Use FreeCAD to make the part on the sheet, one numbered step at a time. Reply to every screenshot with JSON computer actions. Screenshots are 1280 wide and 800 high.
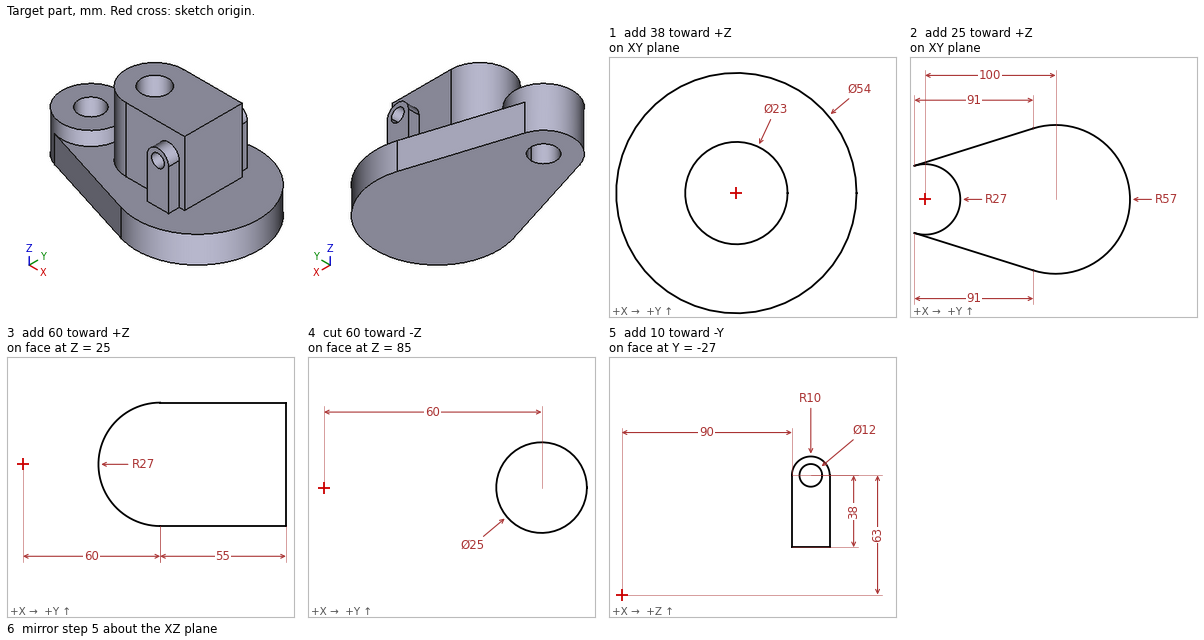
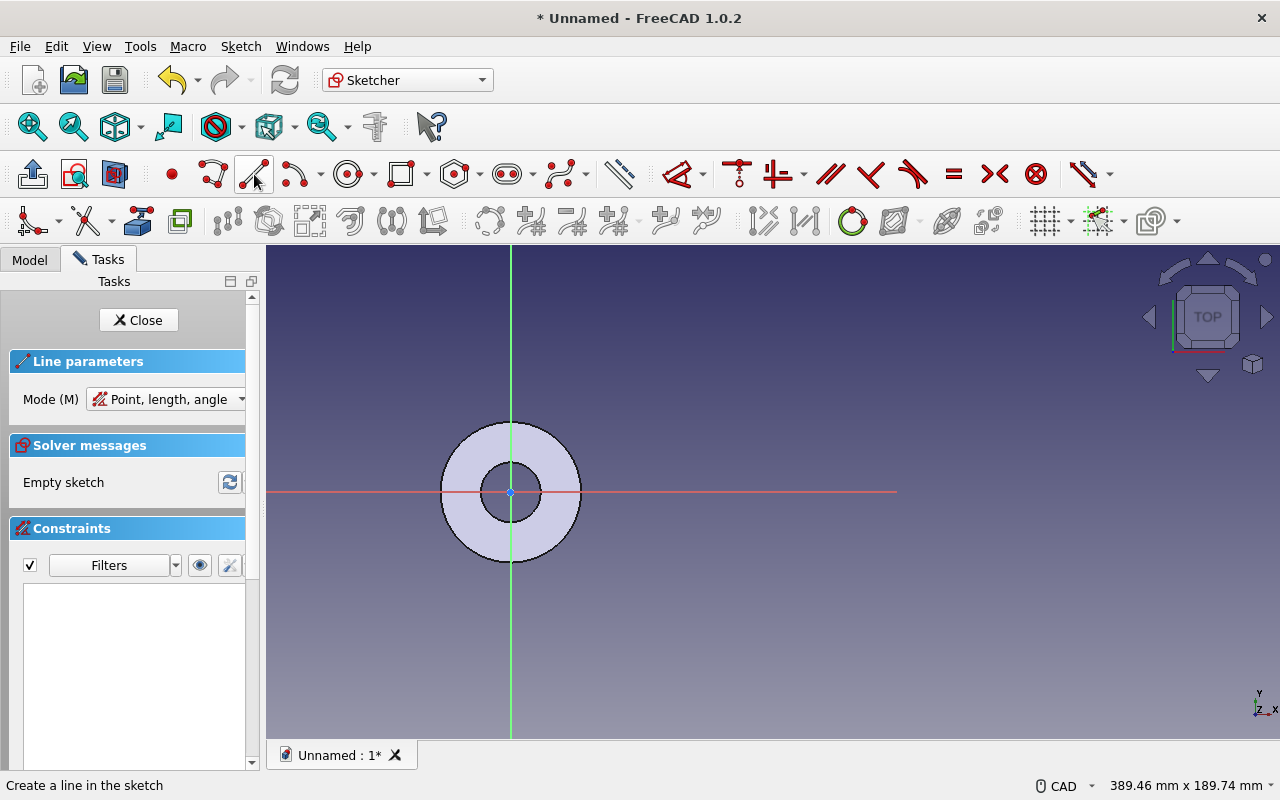
{"action": "left_click", "coordinate": [727, 351]}
{"action": "left_click", "coordinate": [490, 425]}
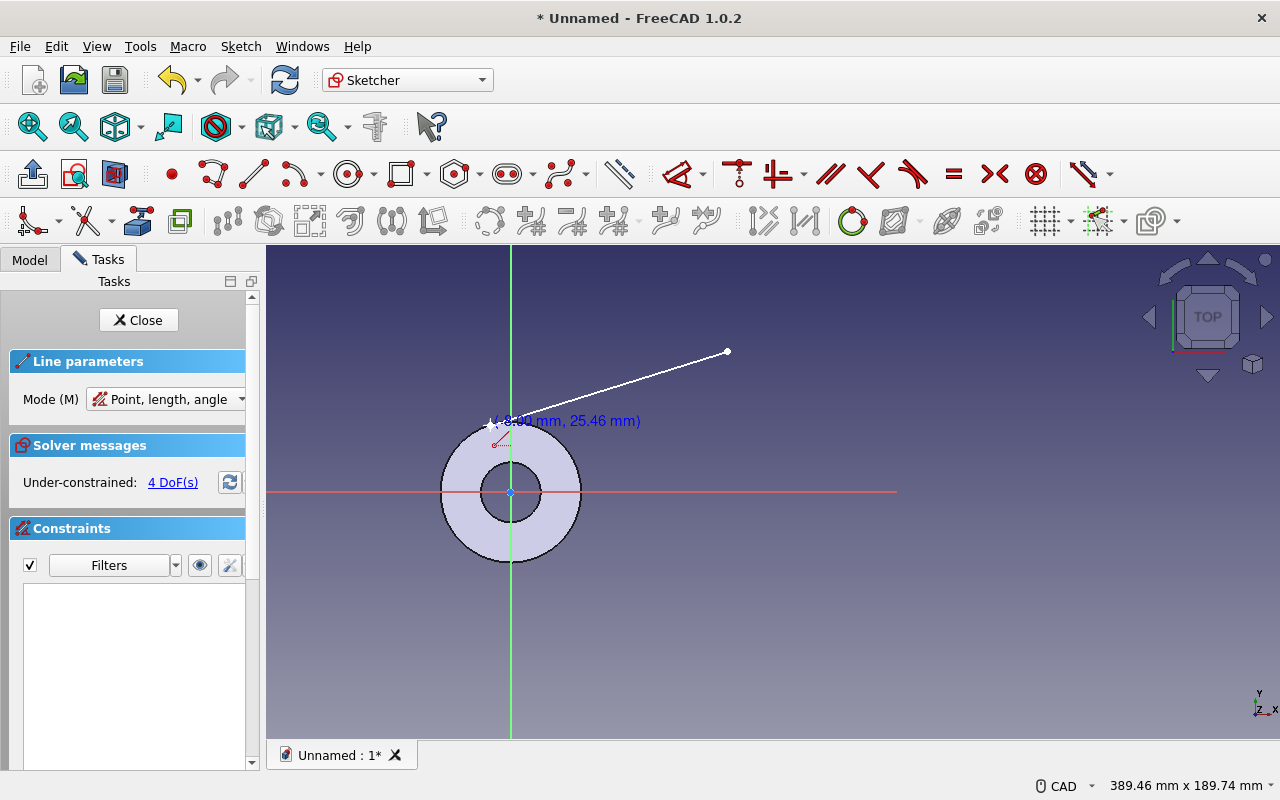
{"action": "left_click", "coordinate": [490, 559]}
{"action": "left_click", "coordinate": [727, 634]}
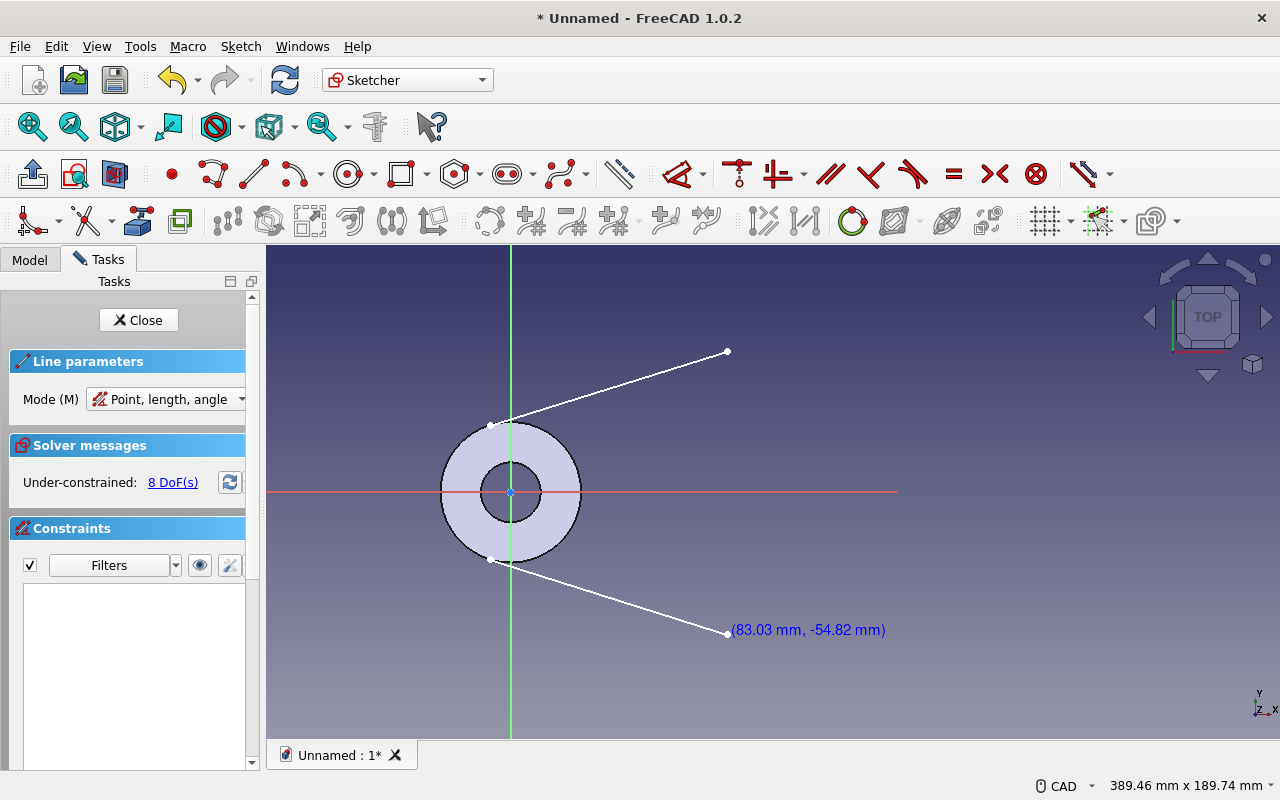
{"action": "left_click", "coordinate": [320, 174]}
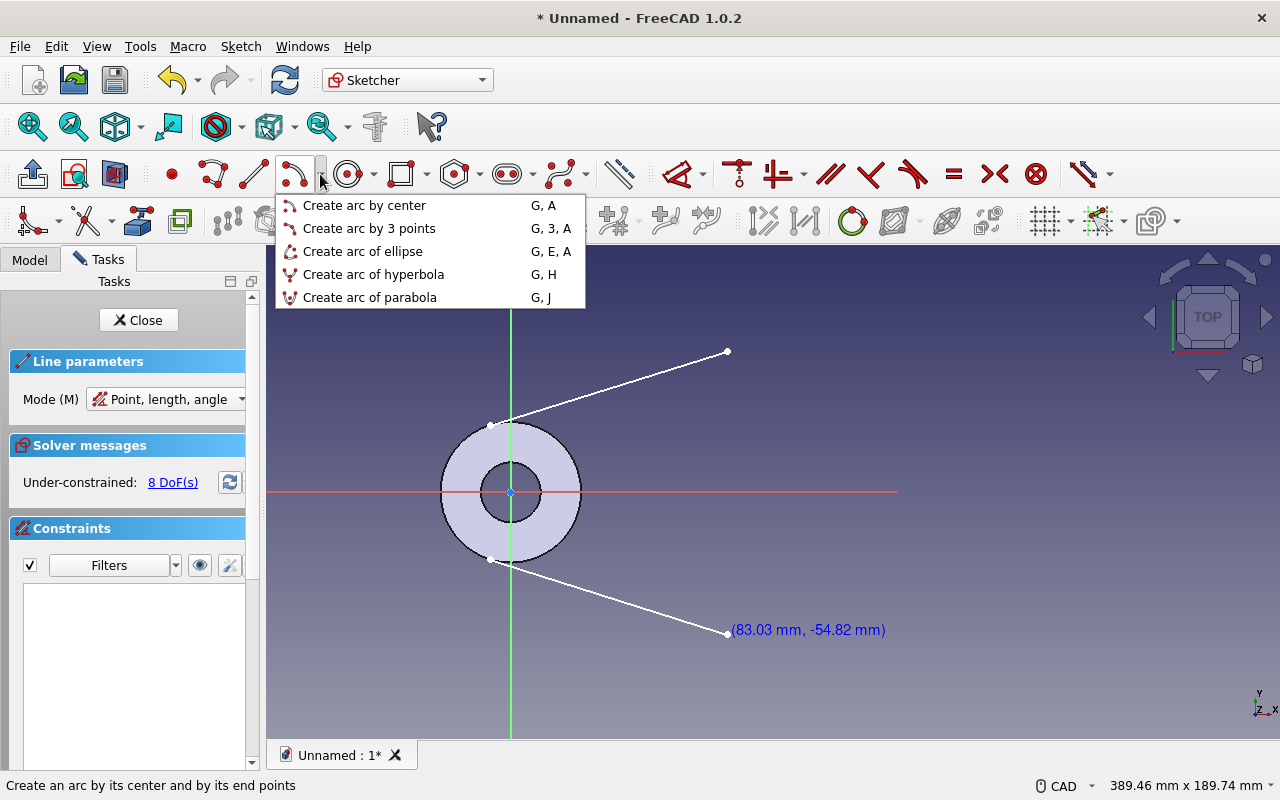
{"action": "left_click", "coordinate": [430, 228]}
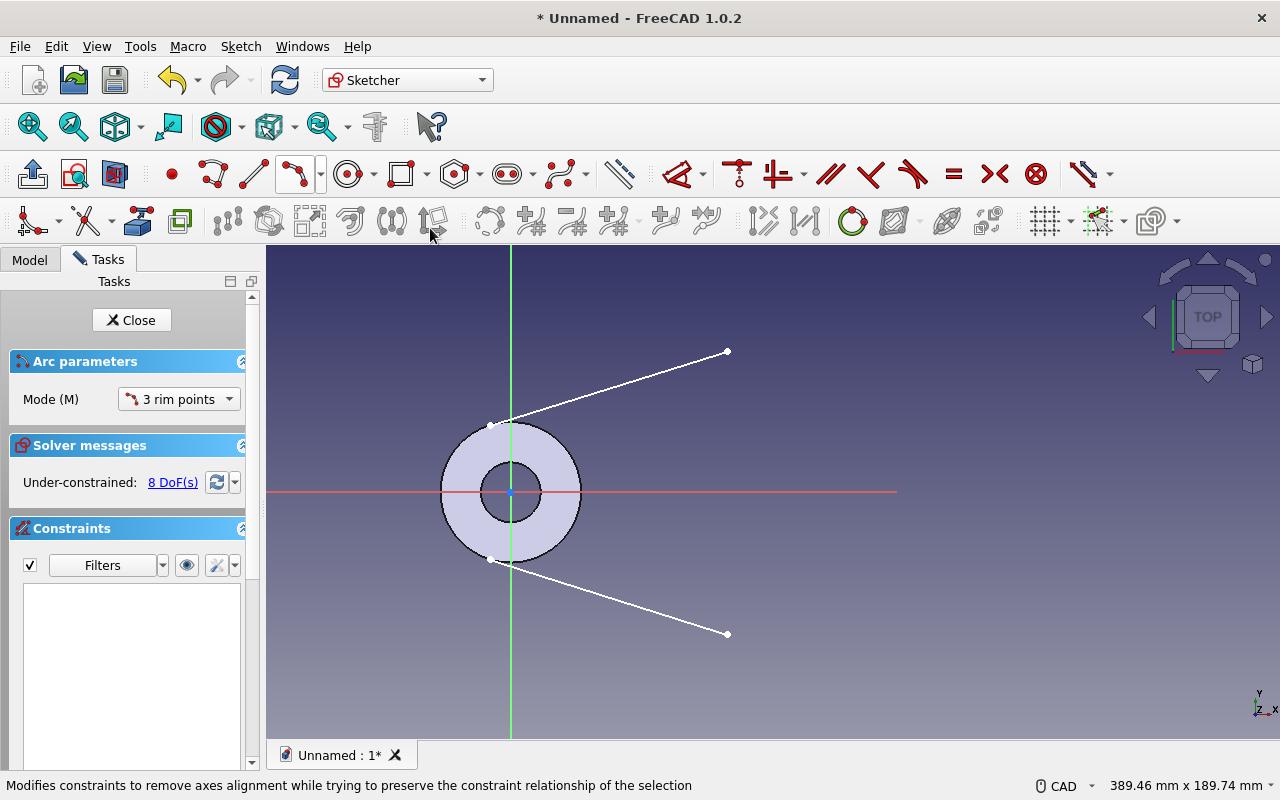
{"action": "left_click", "coordinate": [490, 426]}
{"action": "left_click", "coordinate": [490, 560]}
{"action": "left_click", "coordinate": [576, 518]}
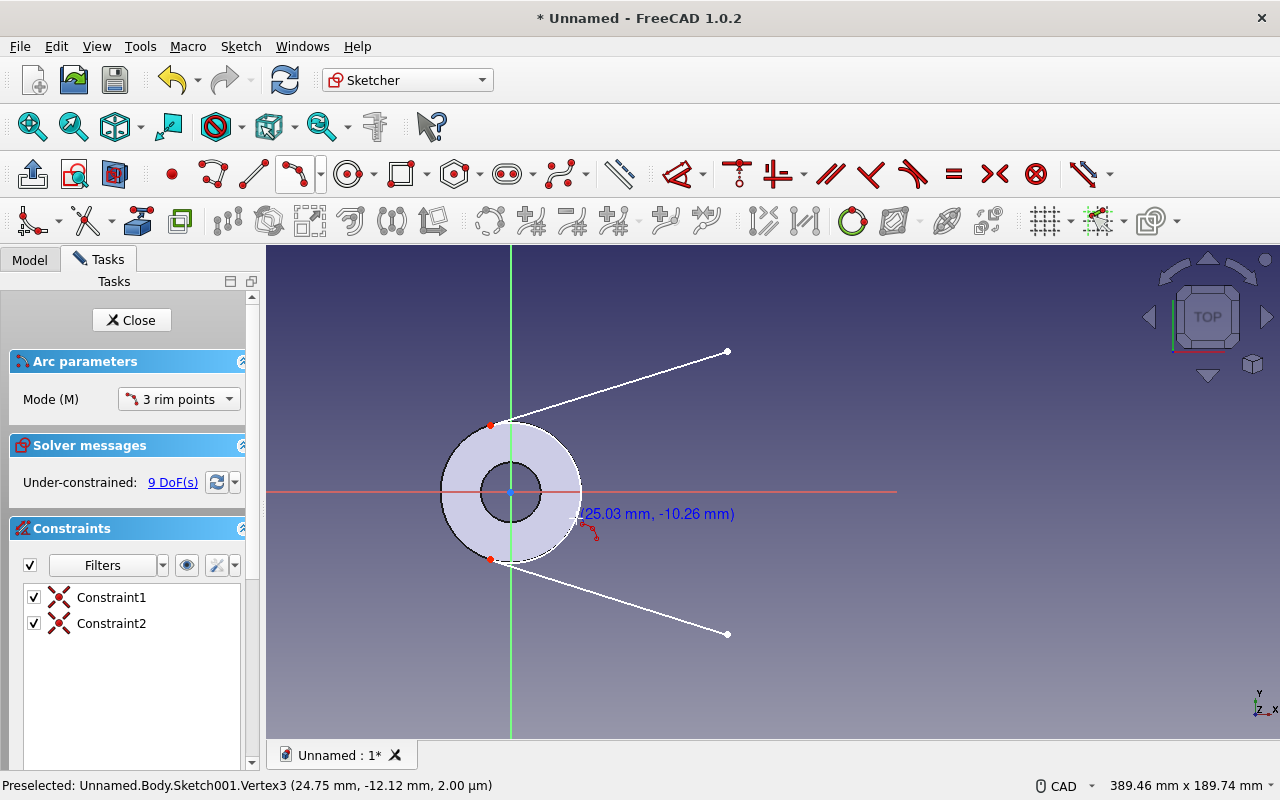
{"action": "left_click", "coordinate": [727, 635]}
{"action": "left_click", "coordinate": [727, 352]}
{"action": "left_click", "coordinate": [909, 547]}
{"action": "key", "text": "Escape"}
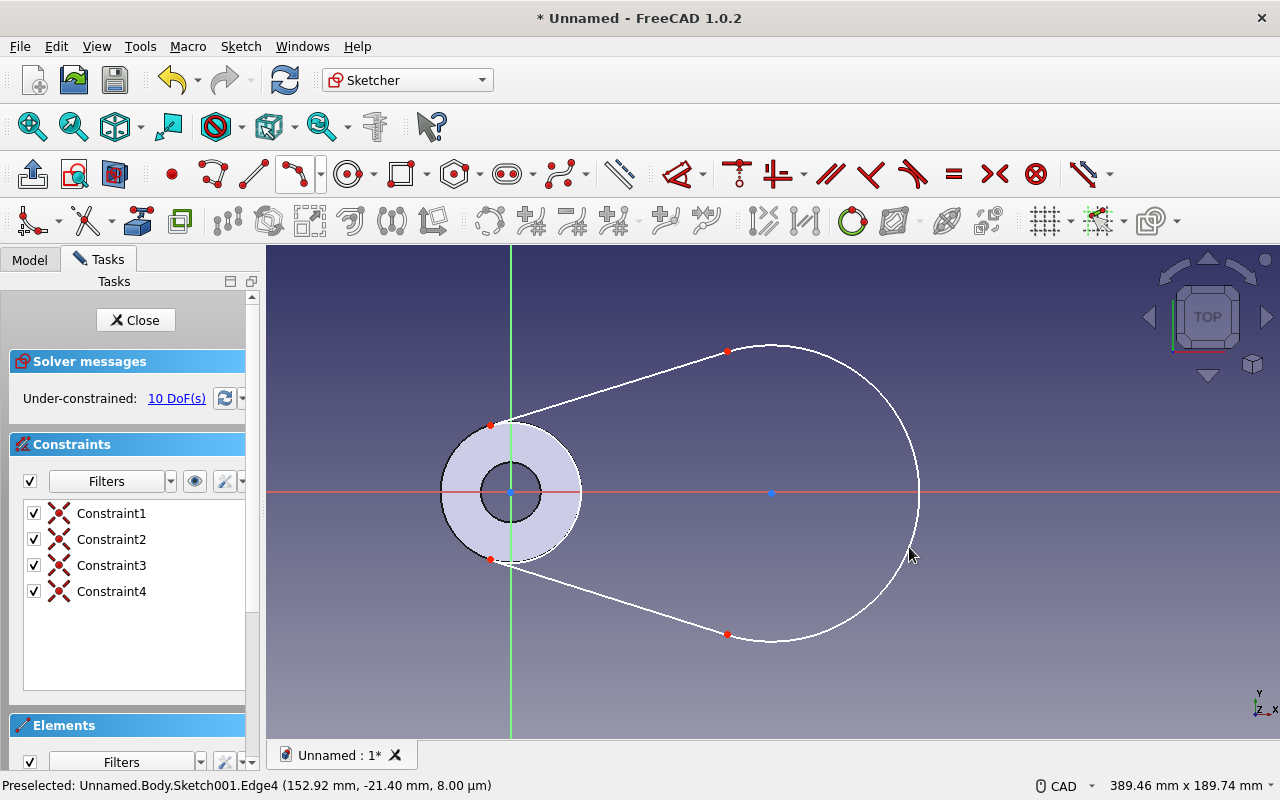
{"action": "left_click", "coordinate": [656, 374]}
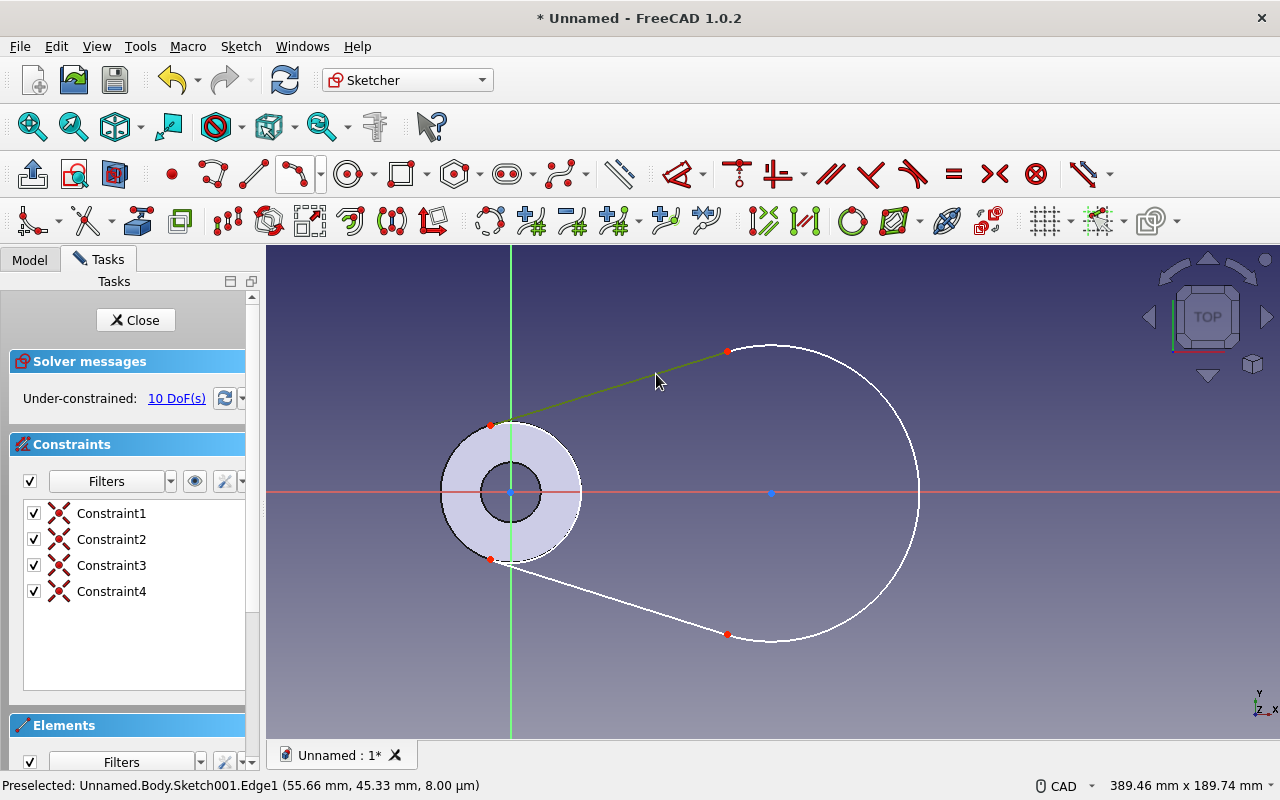
{"action": "left_click", "coordinate": [562, 541]}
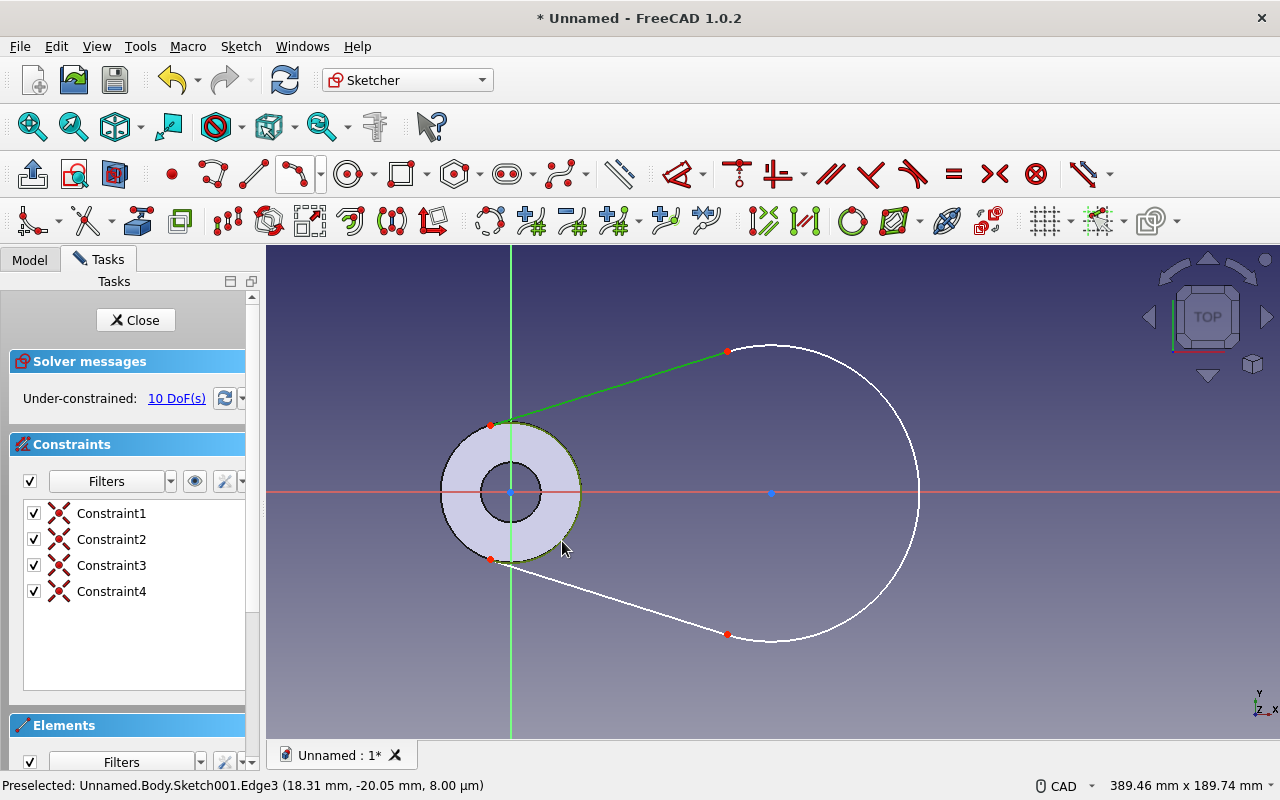
{"action": "left_click", "coordinate": [913, 174]}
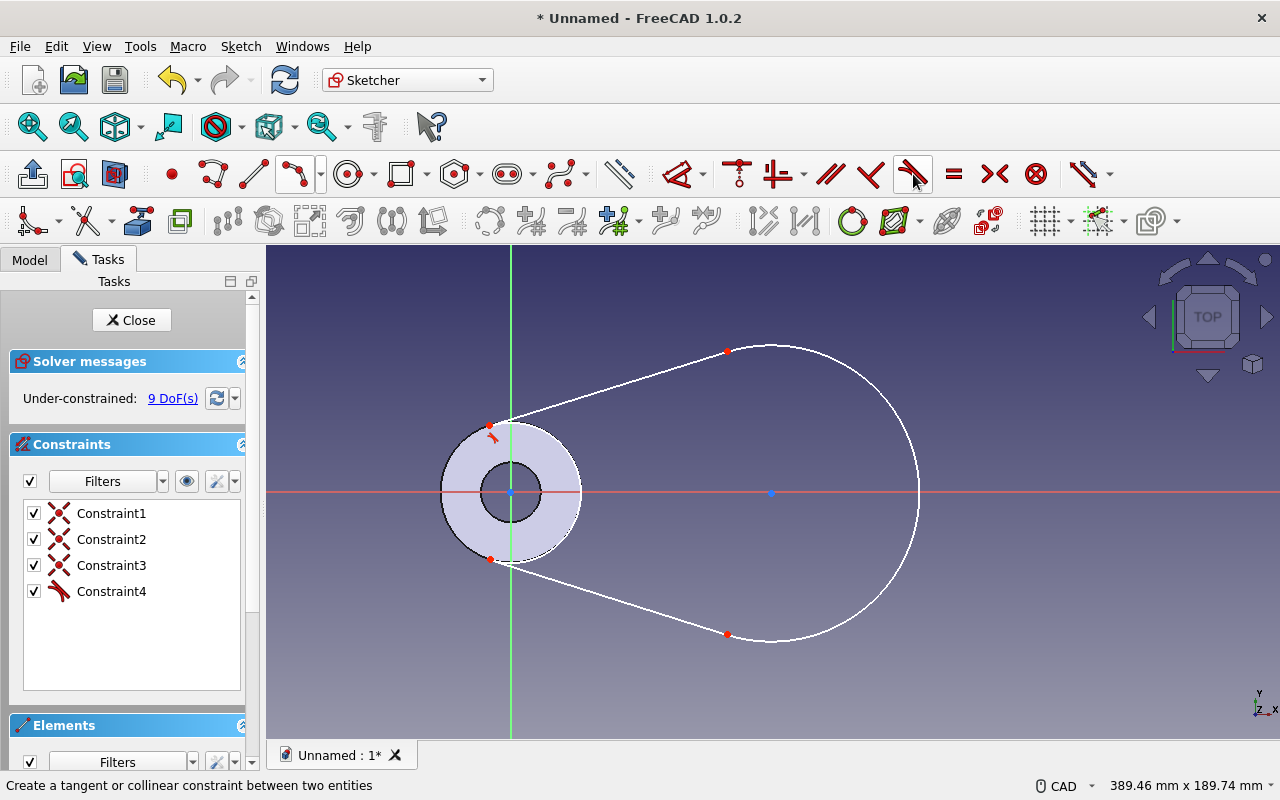
{"action": "left_click", "coordinate": [561, 583]}